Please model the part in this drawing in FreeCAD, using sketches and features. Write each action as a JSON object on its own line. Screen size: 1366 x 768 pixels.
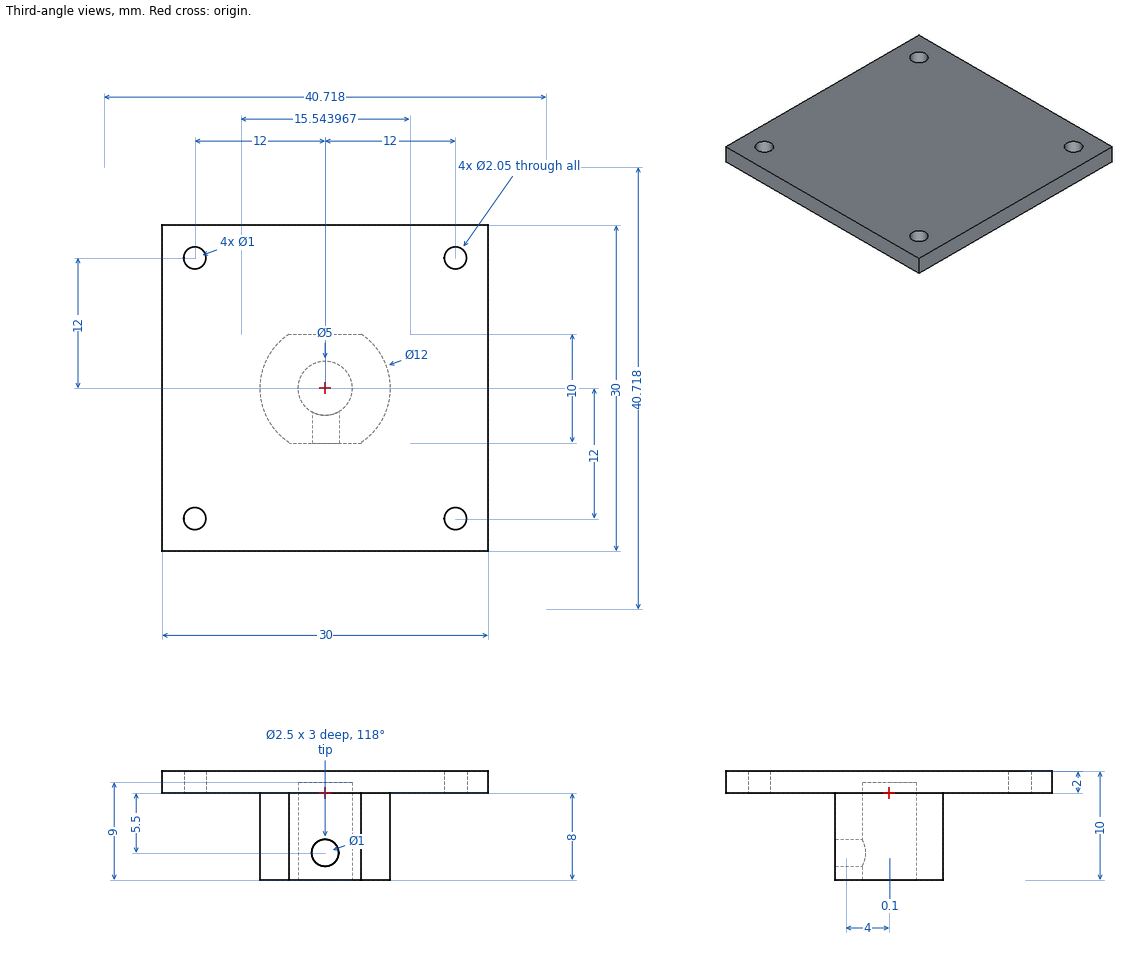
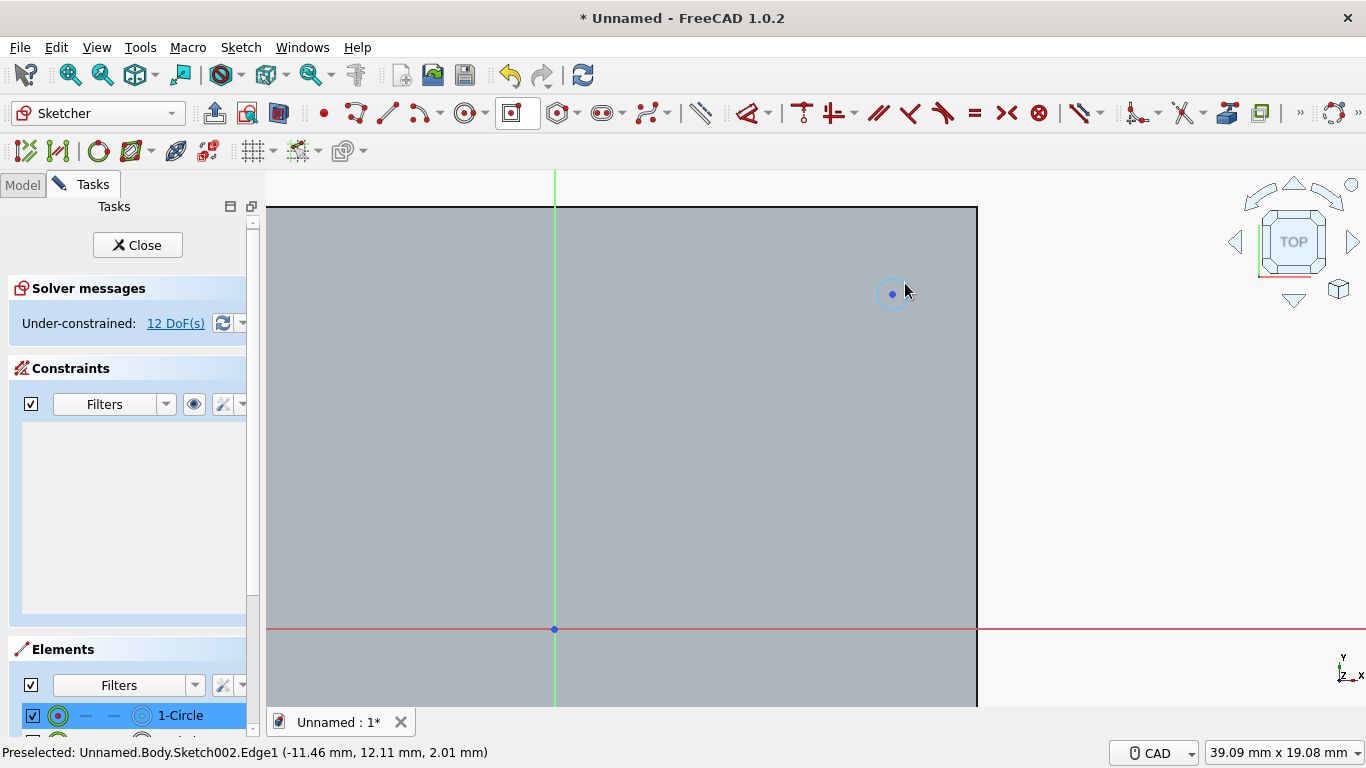
{"action": "left_click", "coordinate": [904, 283]}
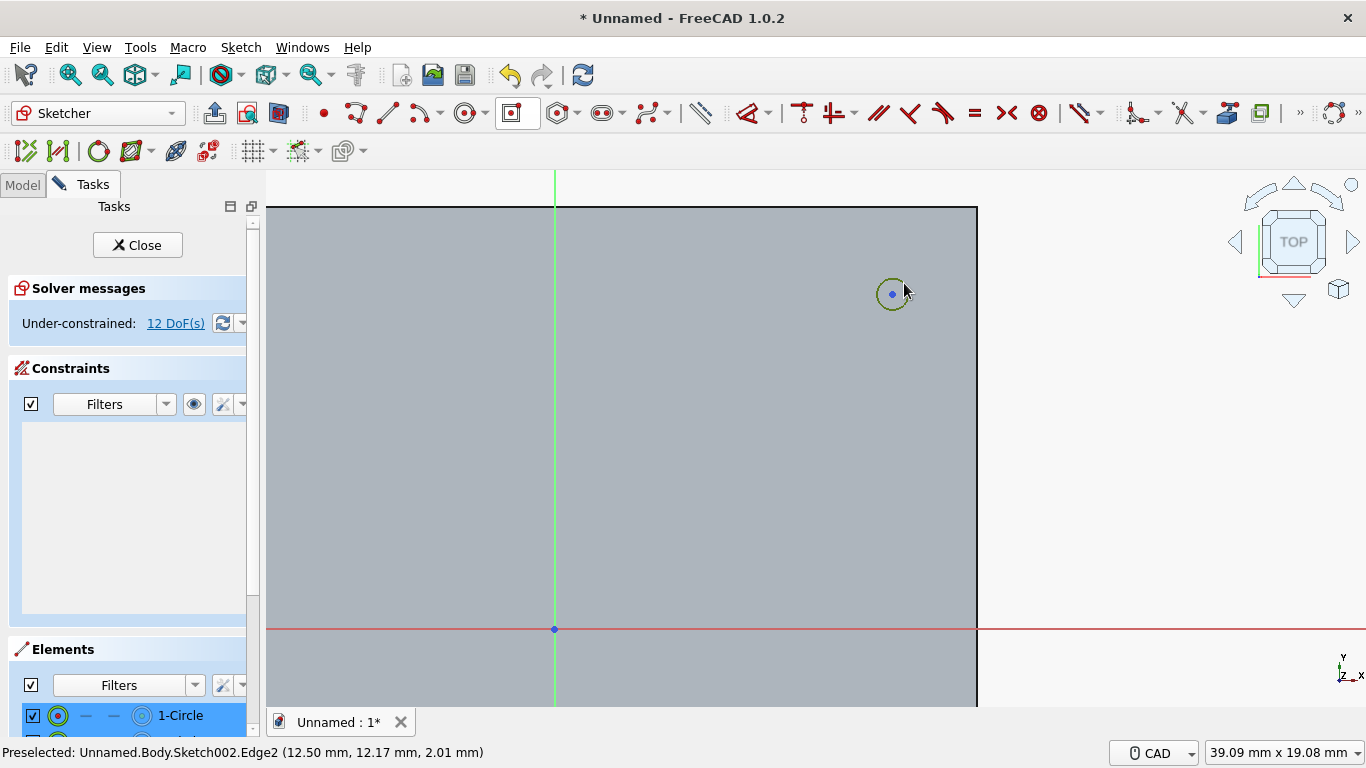
{"action": "scroll", "coordinate": [905, 283], "scroll_direction": "down", "scroll_amount": 4}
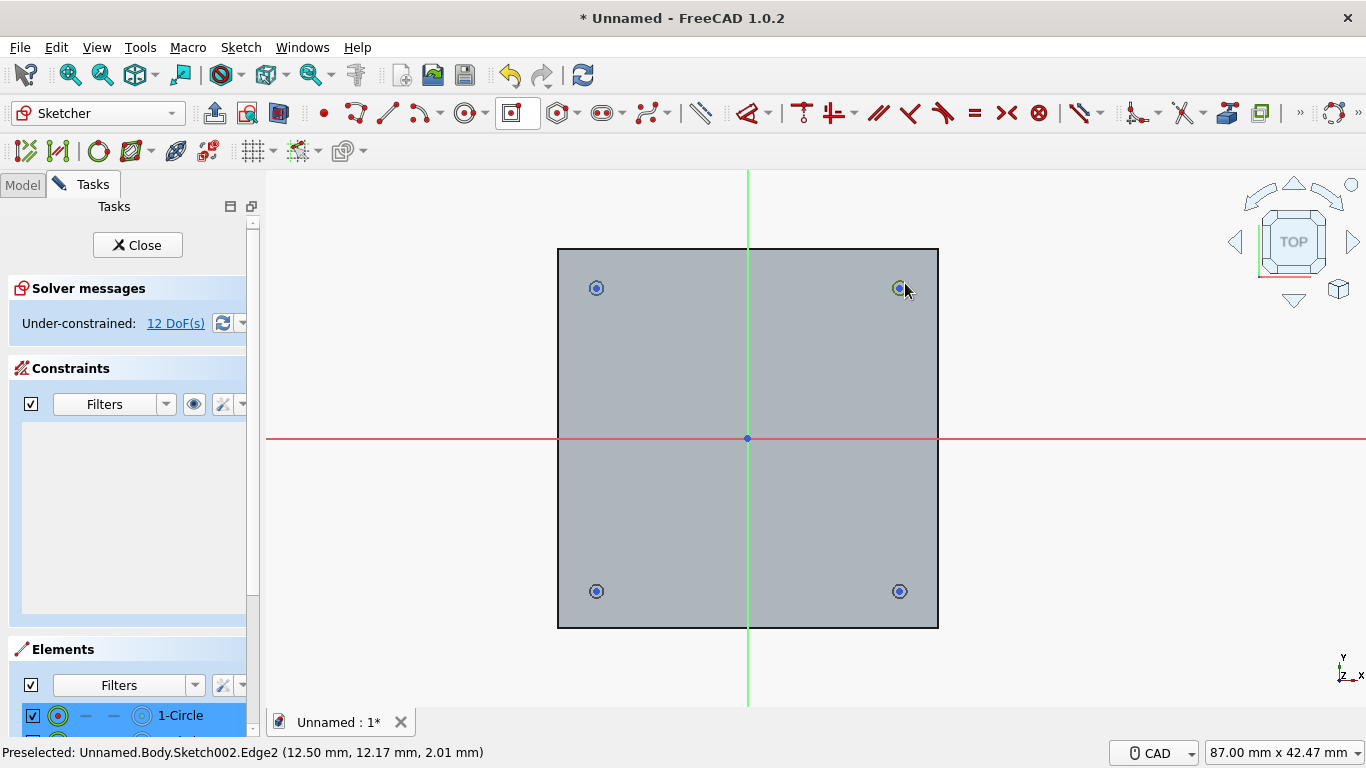
{"action": "scroll", "coordinate": [905, 587], "scroll_direction": "up", "scroll_amount": 4}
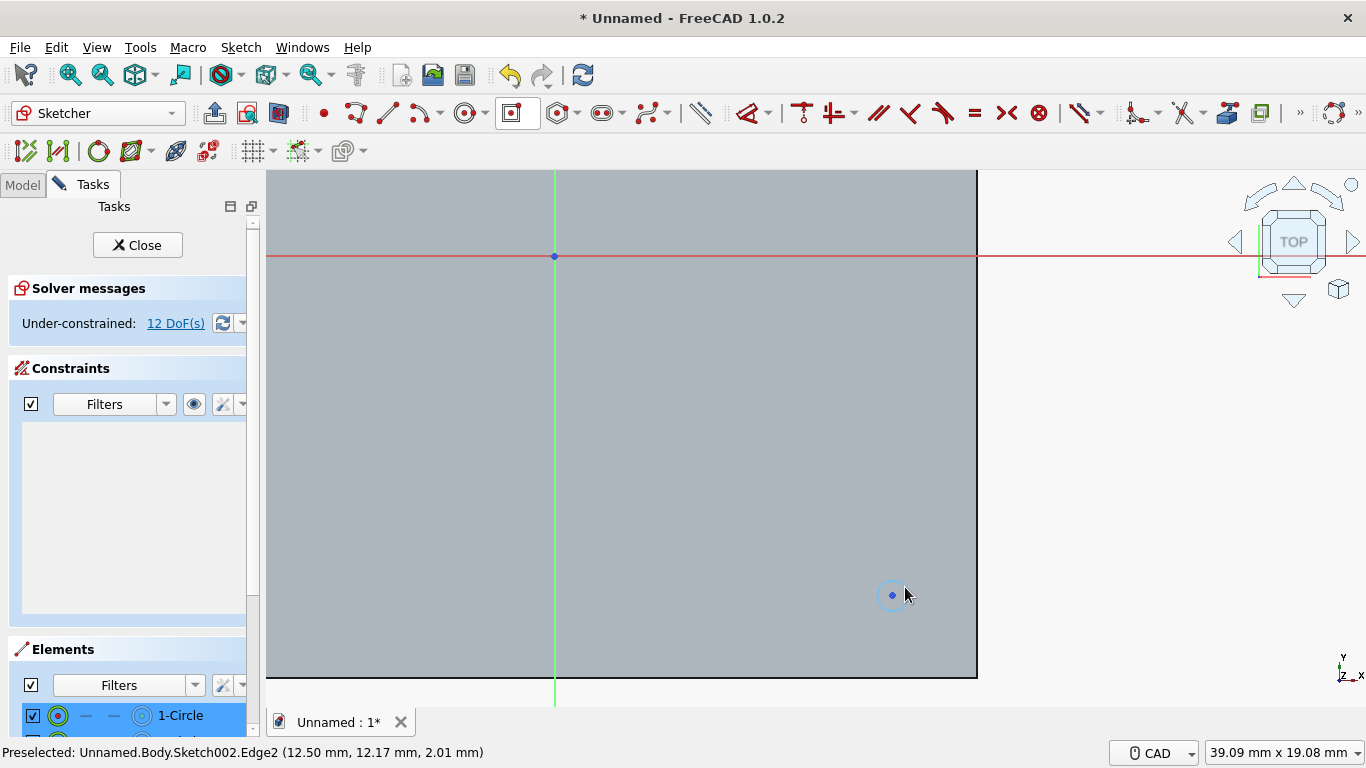
{"action": "left_click", "coordinate": [903, 585]}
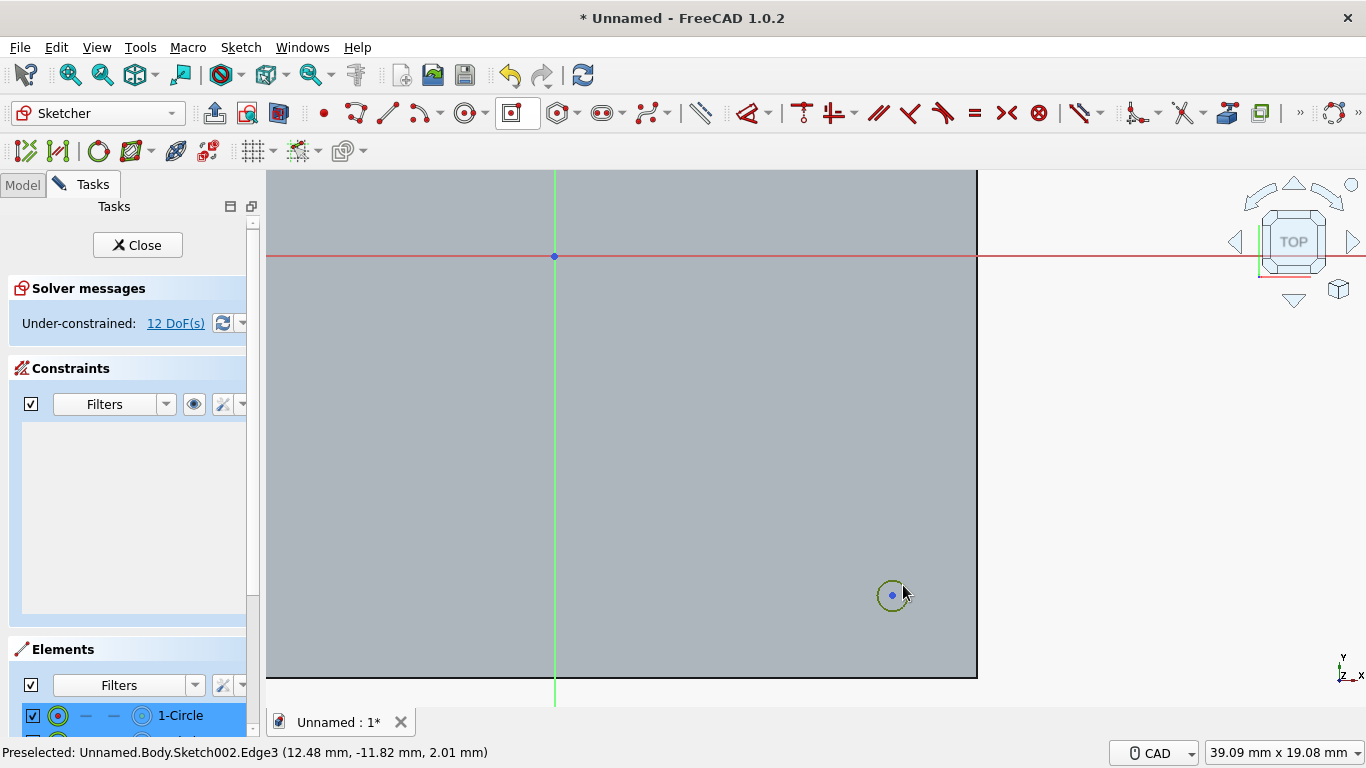
{"action": "scroll", "coordinate": [905, 587], "scroll_direction": "down", "scroll_amount": 4}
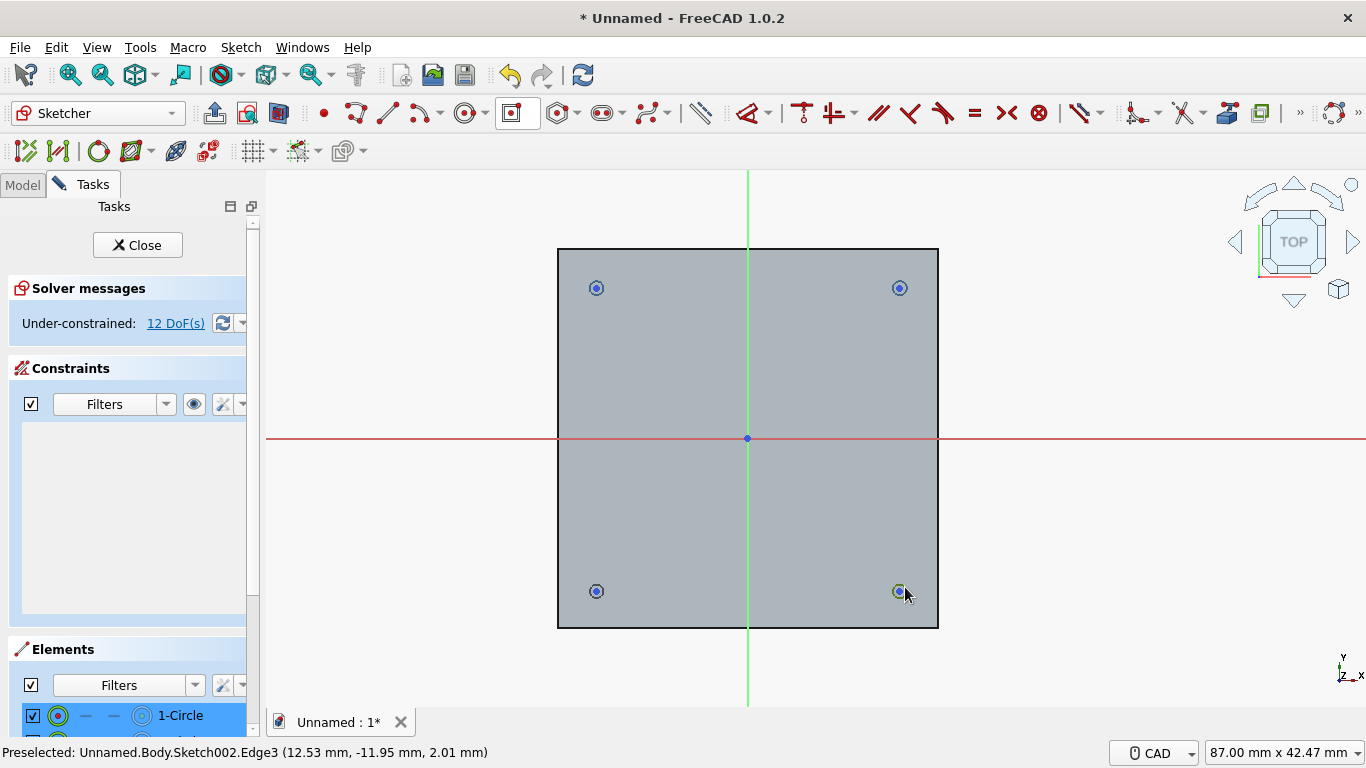
{"action": "scroll", "coordinate": [601, 587], "scroll_direction": "up", "scroll_amount": 4}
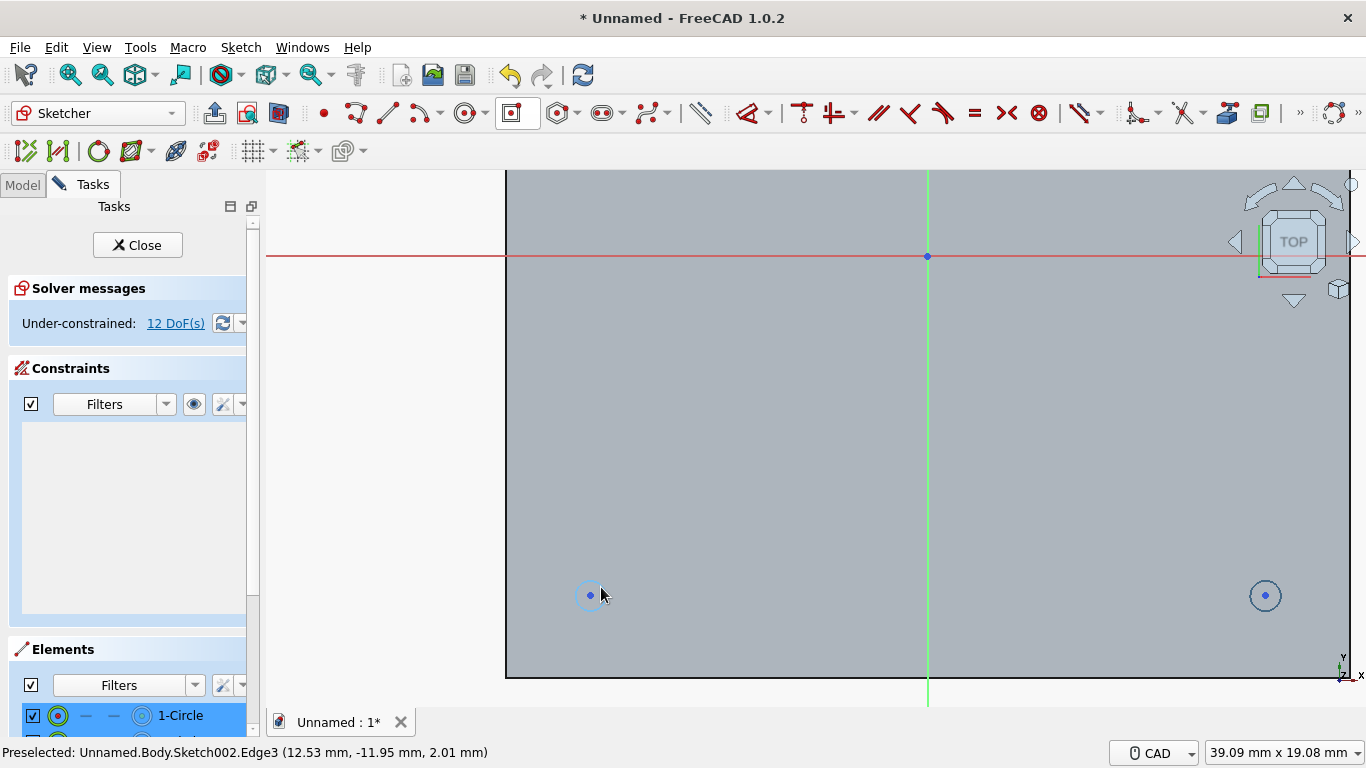
{"action": "left_click", "coordinate": [601, 585]}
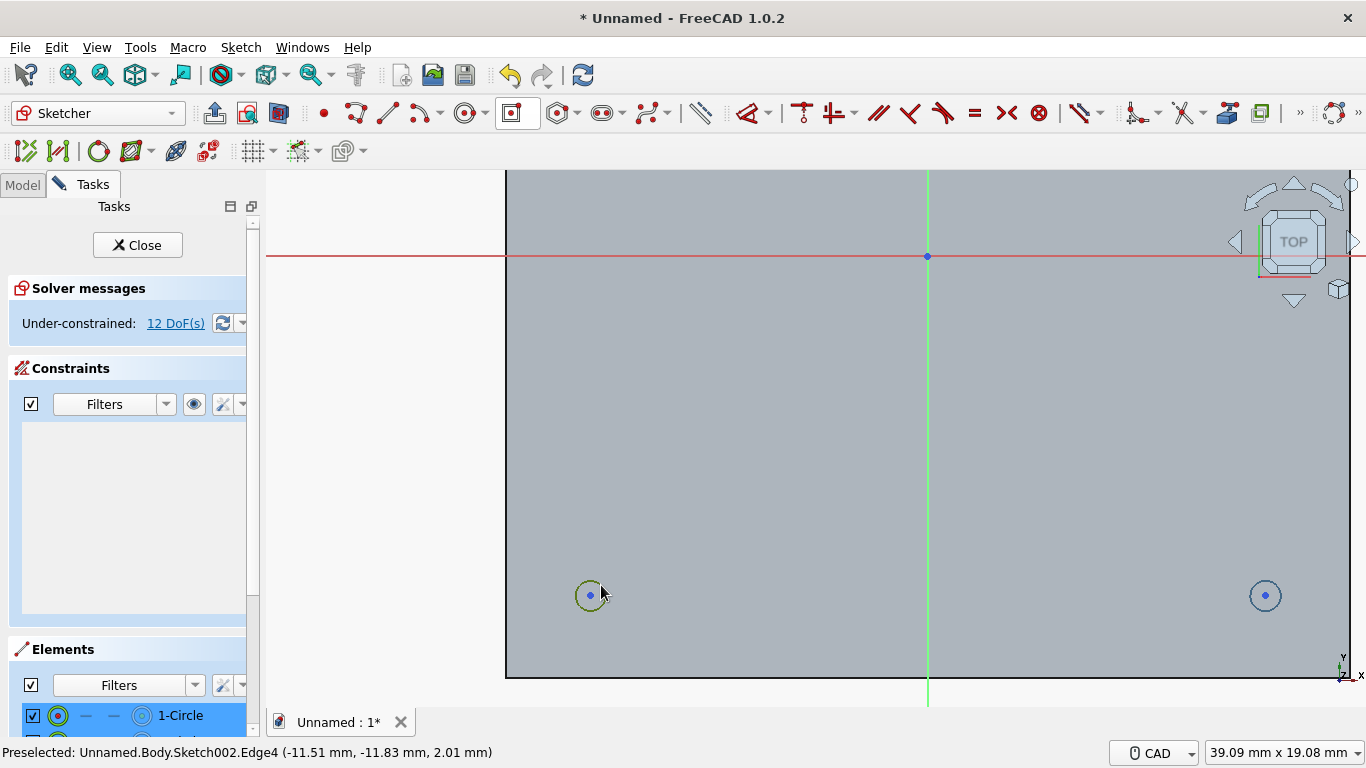
{"action": "key", "text": "e"}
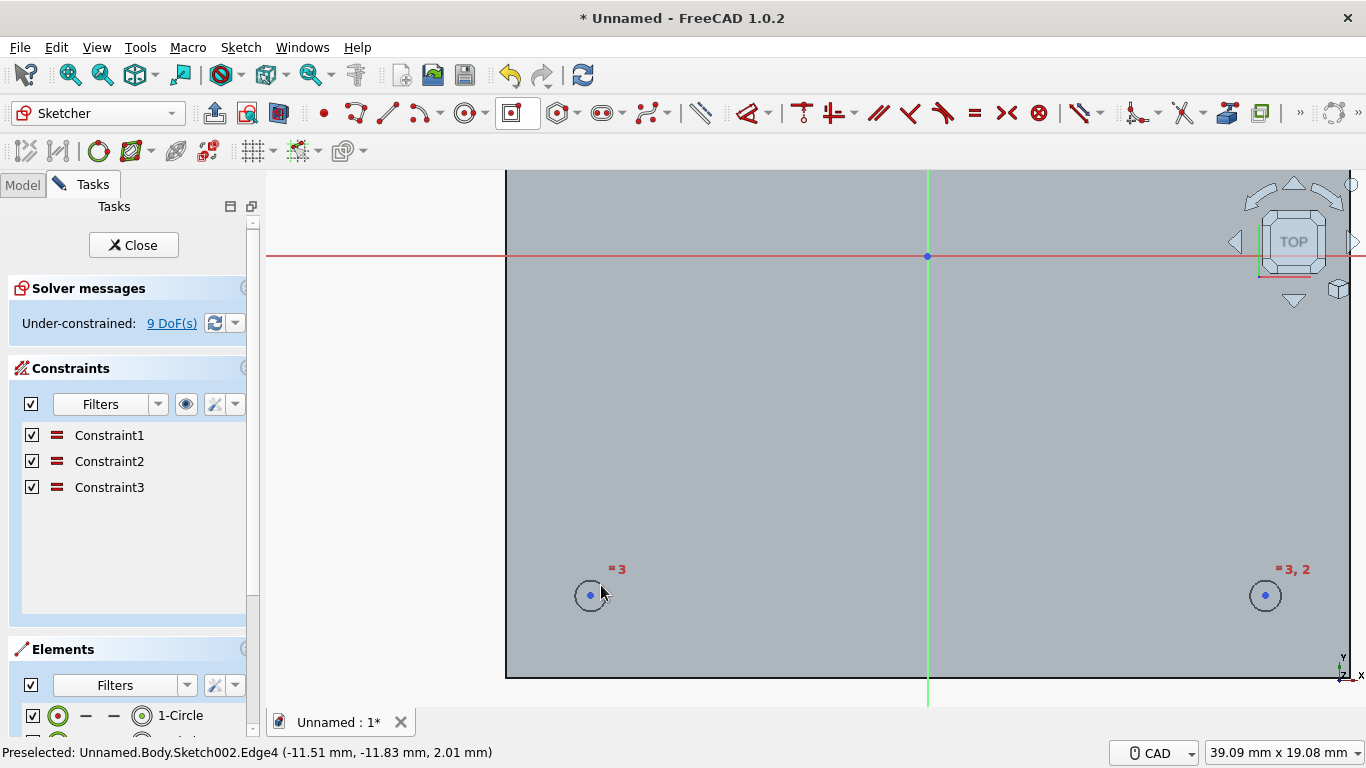
{"action": "scroll", "coordinate": [601, 587], "scroll_direction": "down", "scroll_amount": 4}